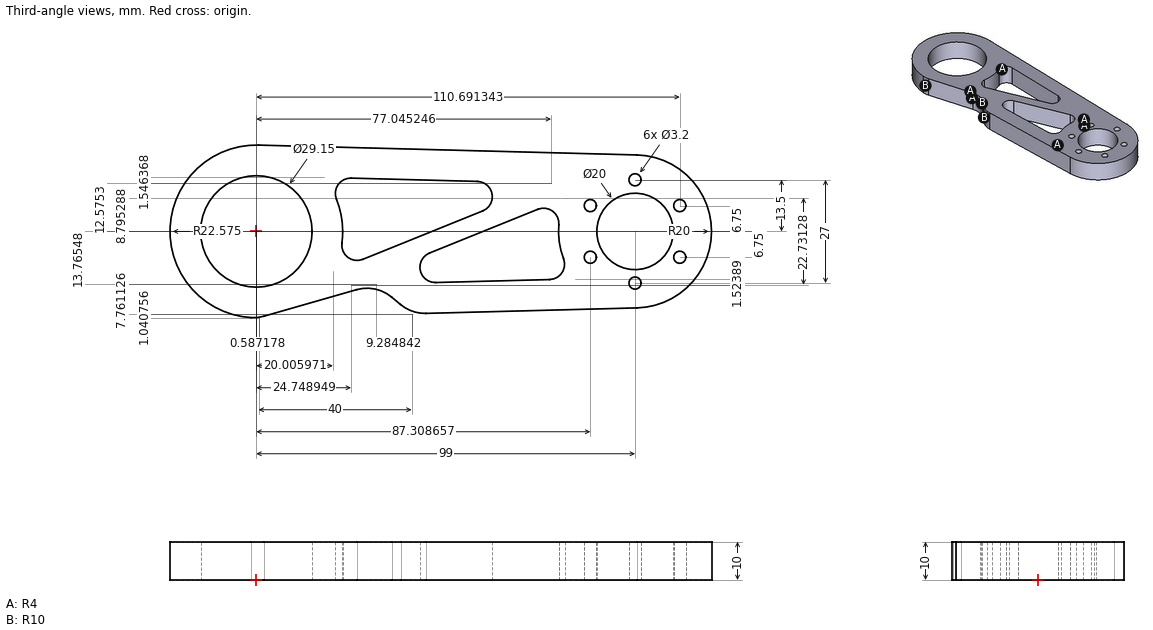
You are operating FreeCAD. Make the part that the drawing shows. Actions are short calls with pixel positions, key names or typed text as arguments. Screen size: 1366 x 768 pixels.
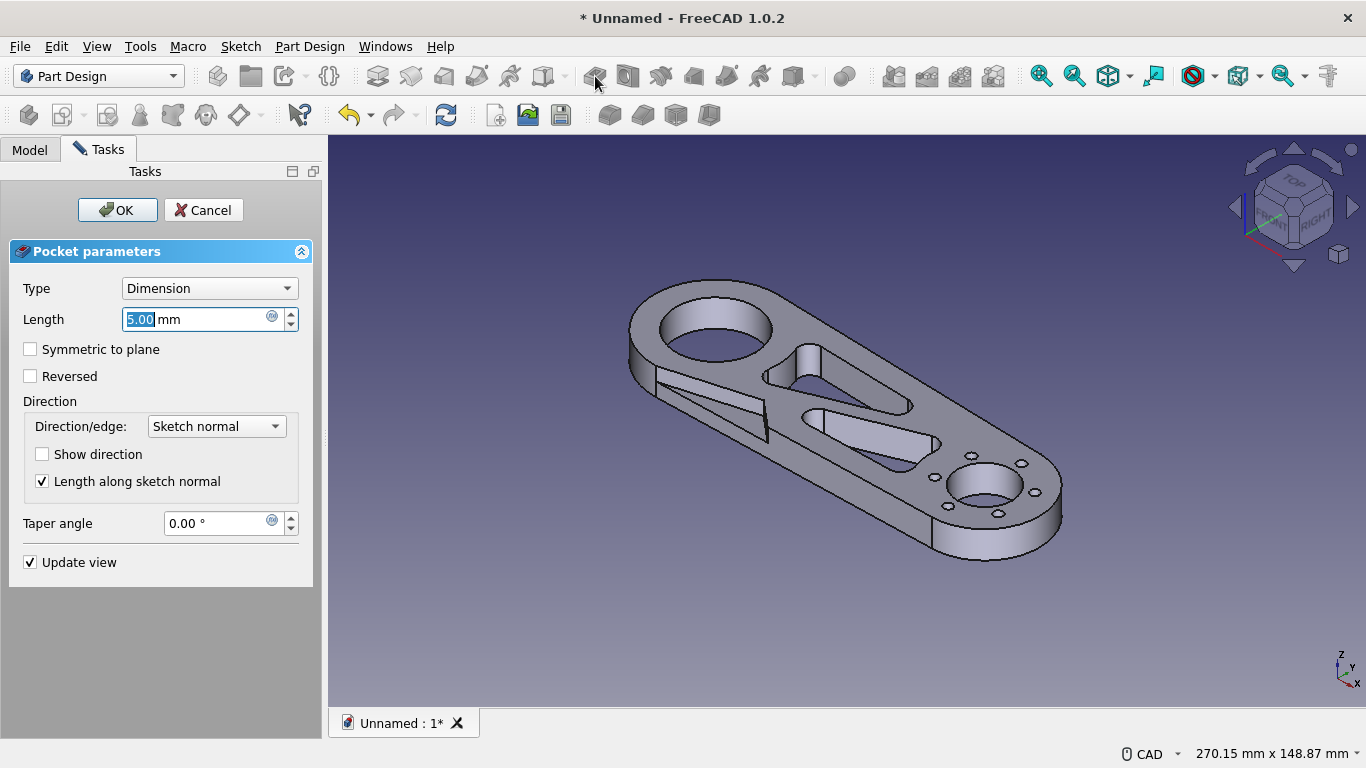
text(10)
key(Tab)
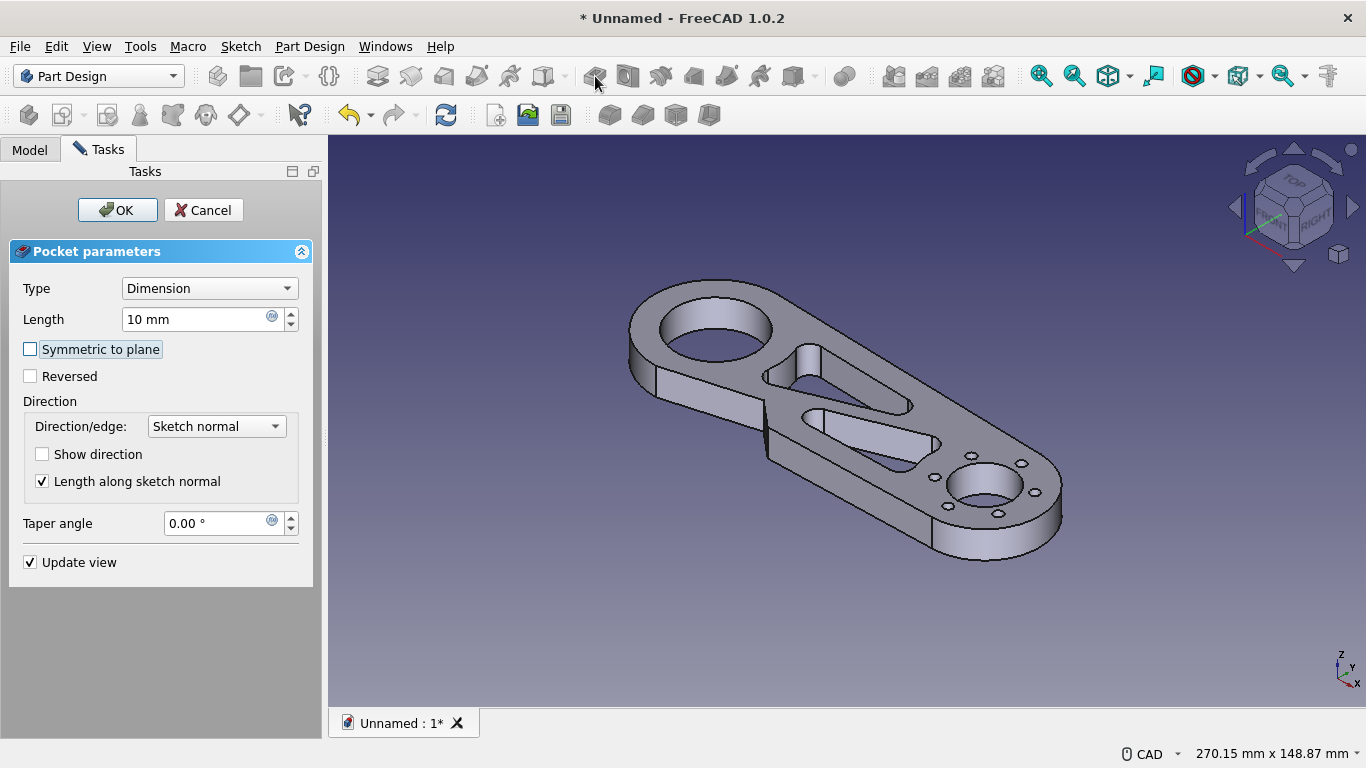
click(118, 210)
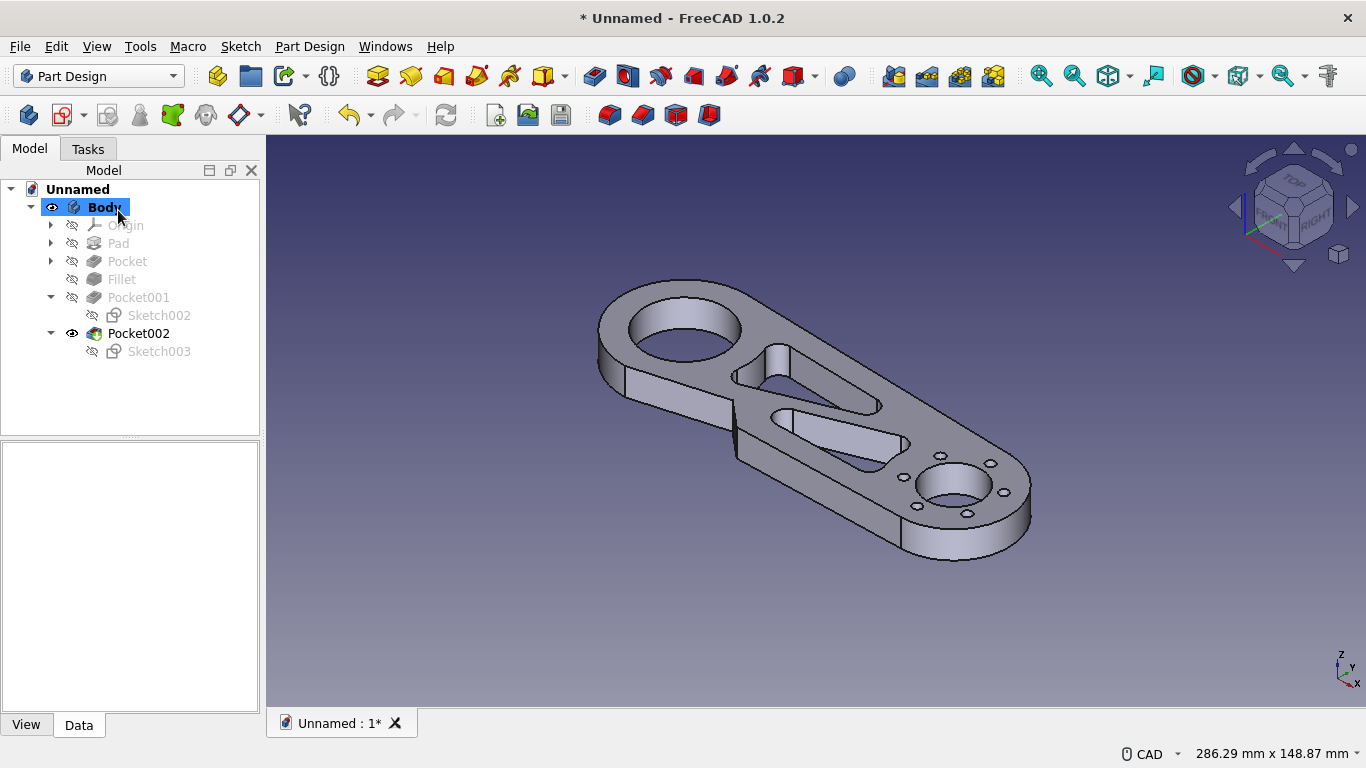
key(2)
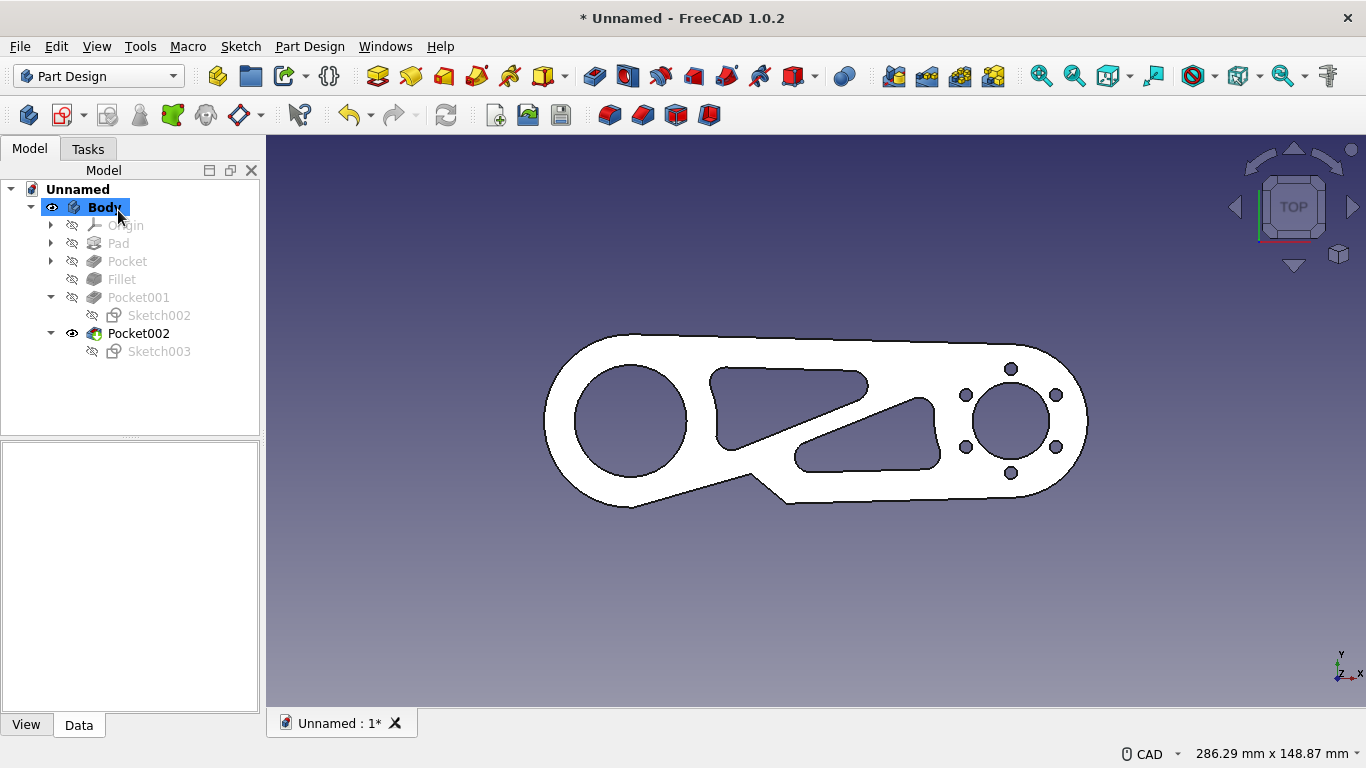
key(0)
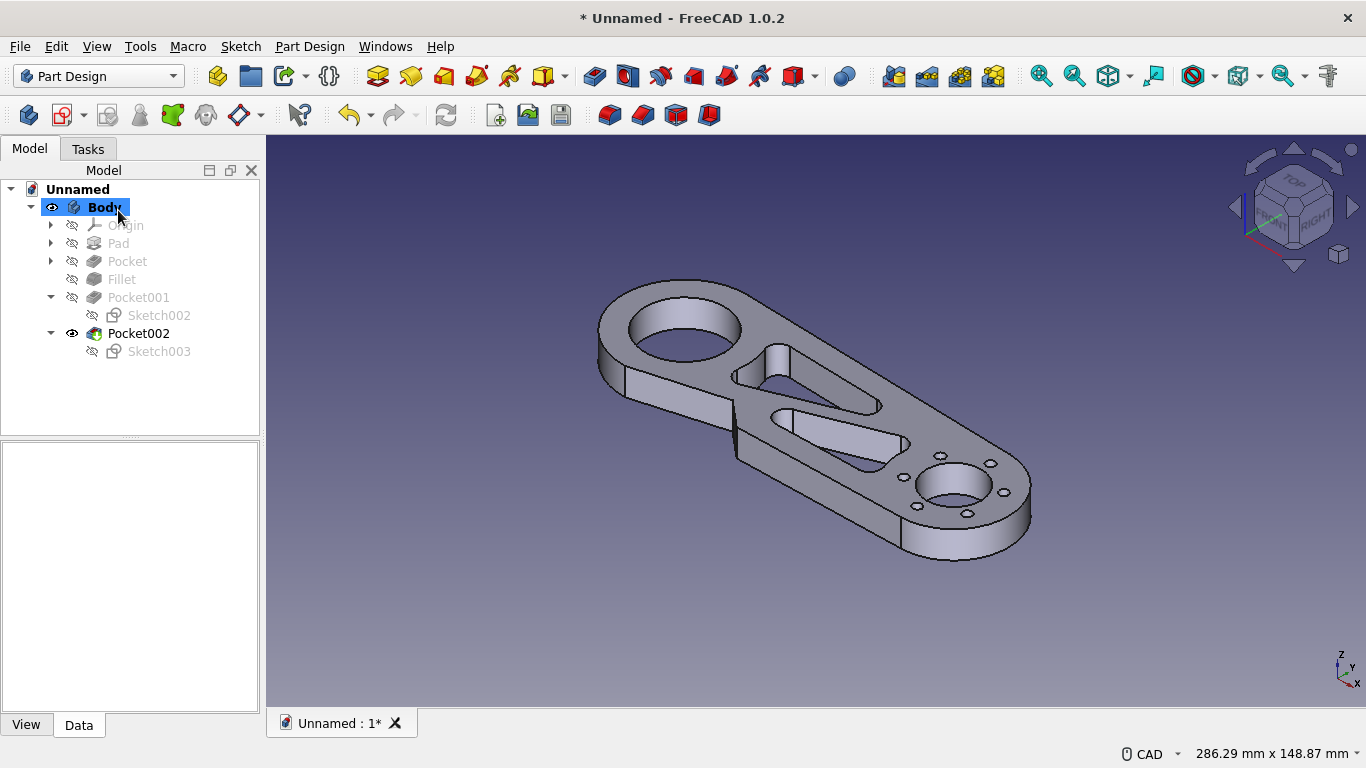
key(1)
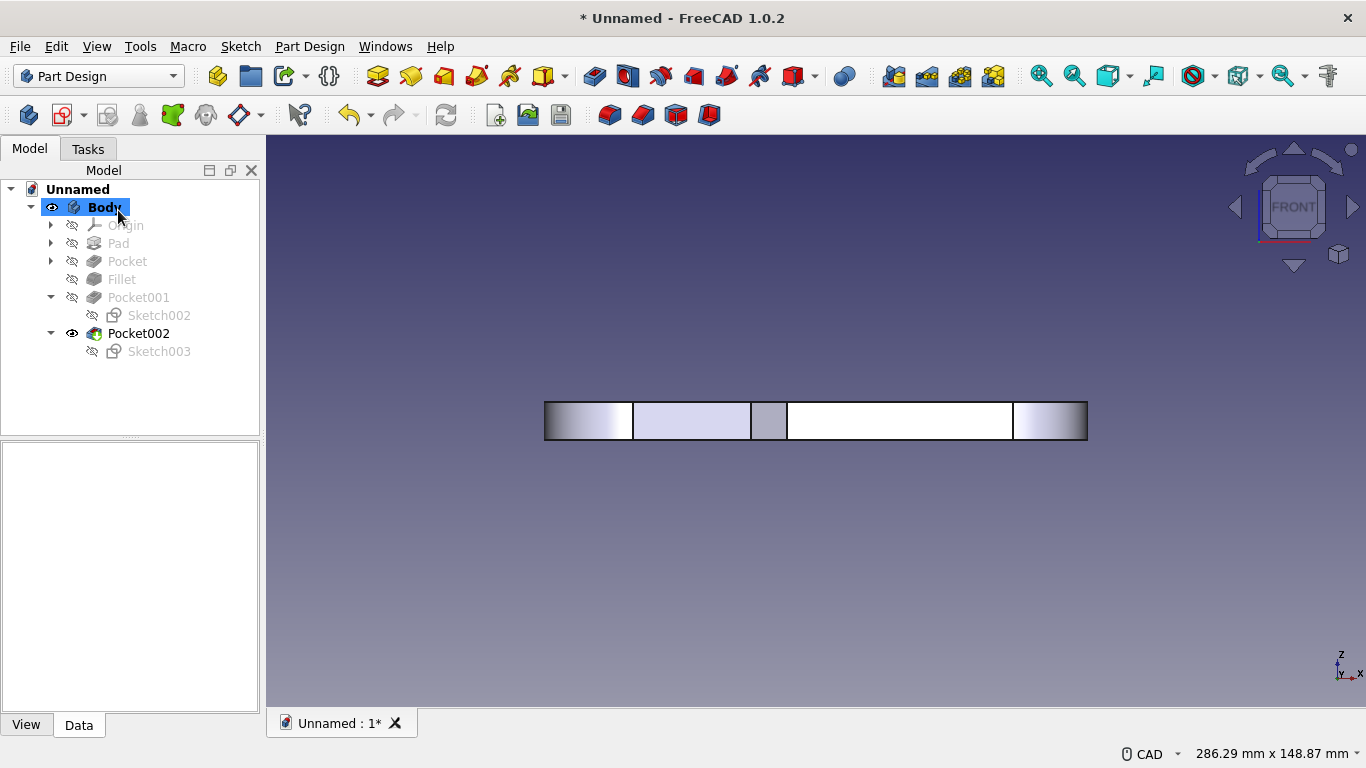
click(633, 420)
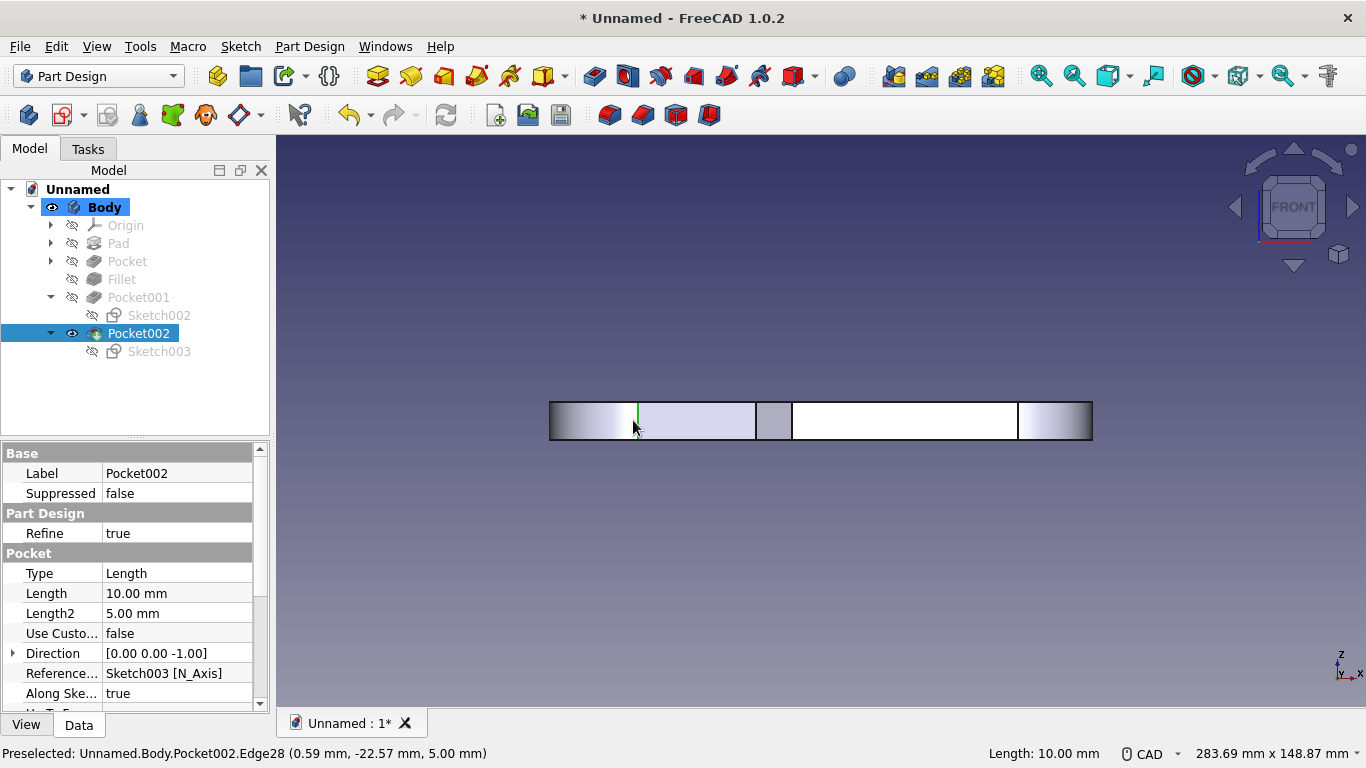
click(792, 420, ctrl)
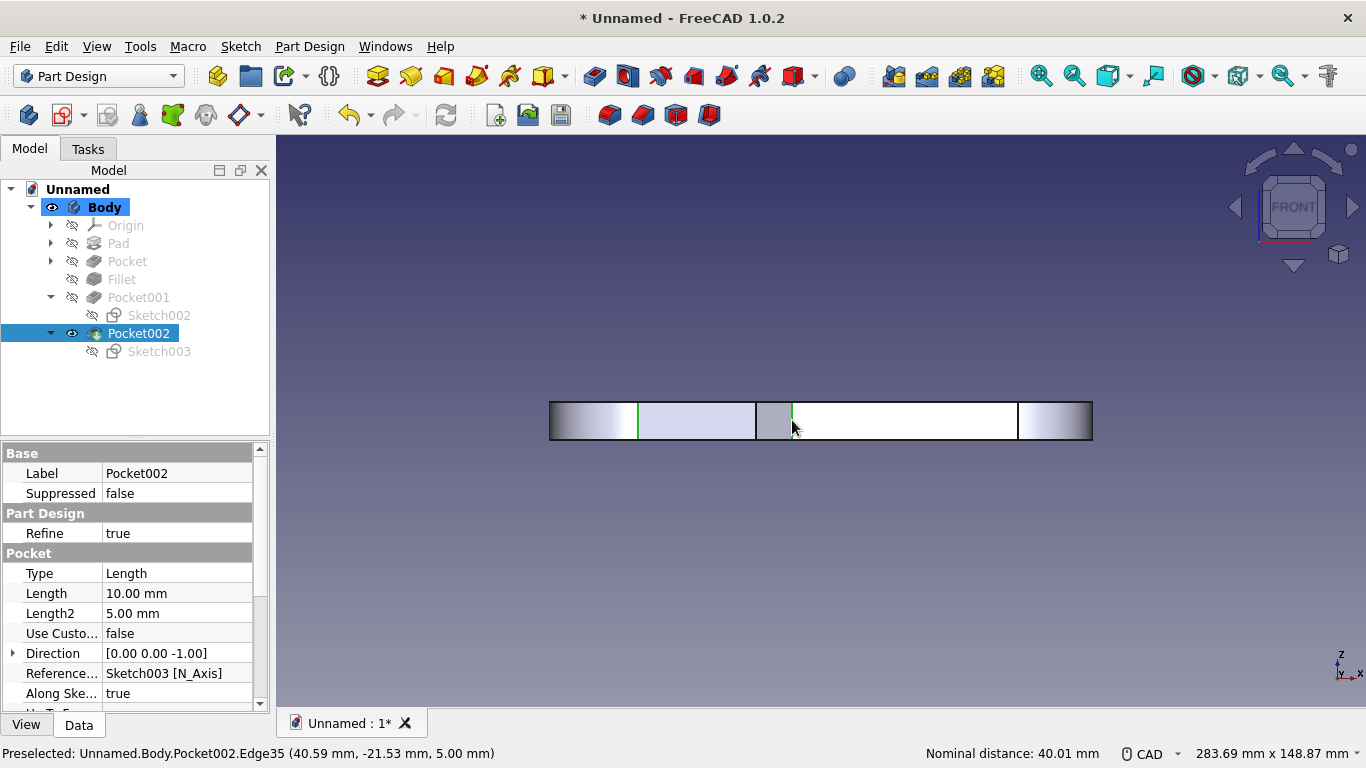
key(3)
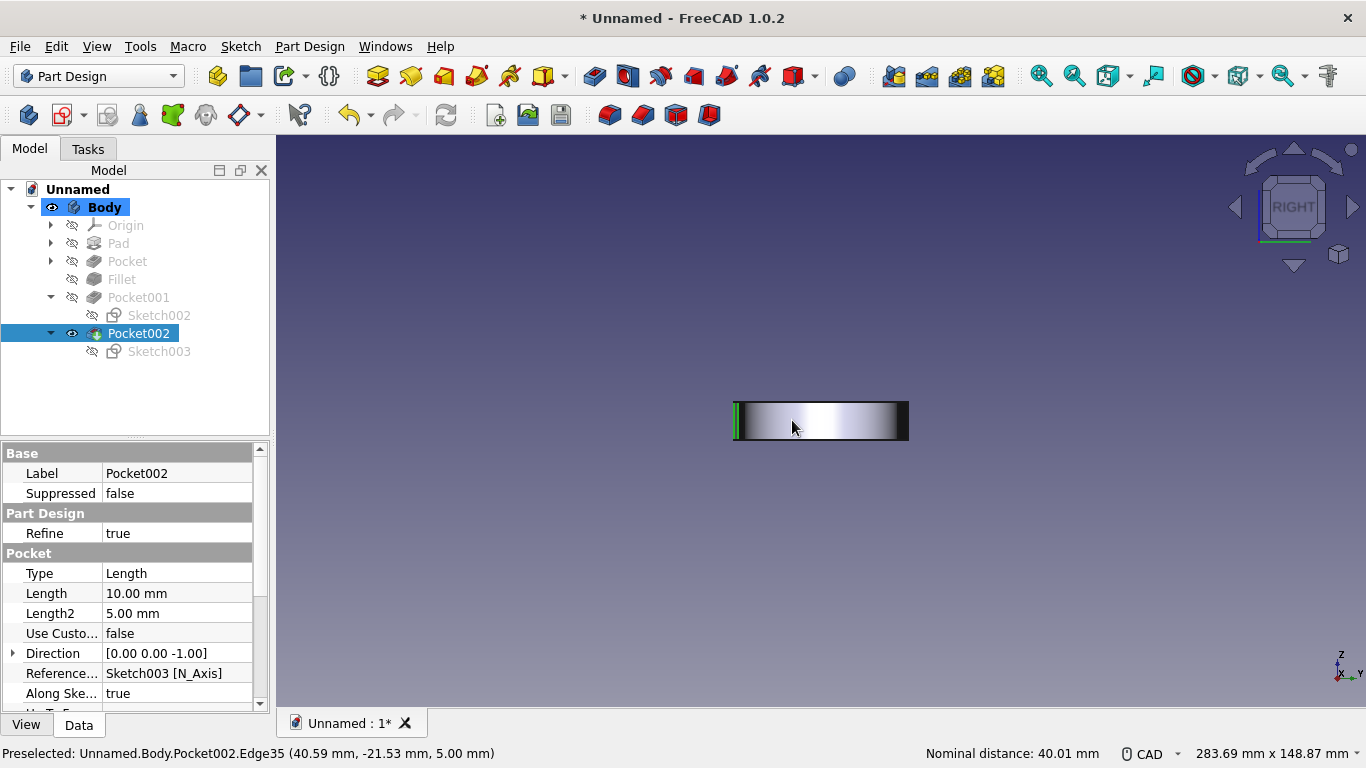
click(1042, 76)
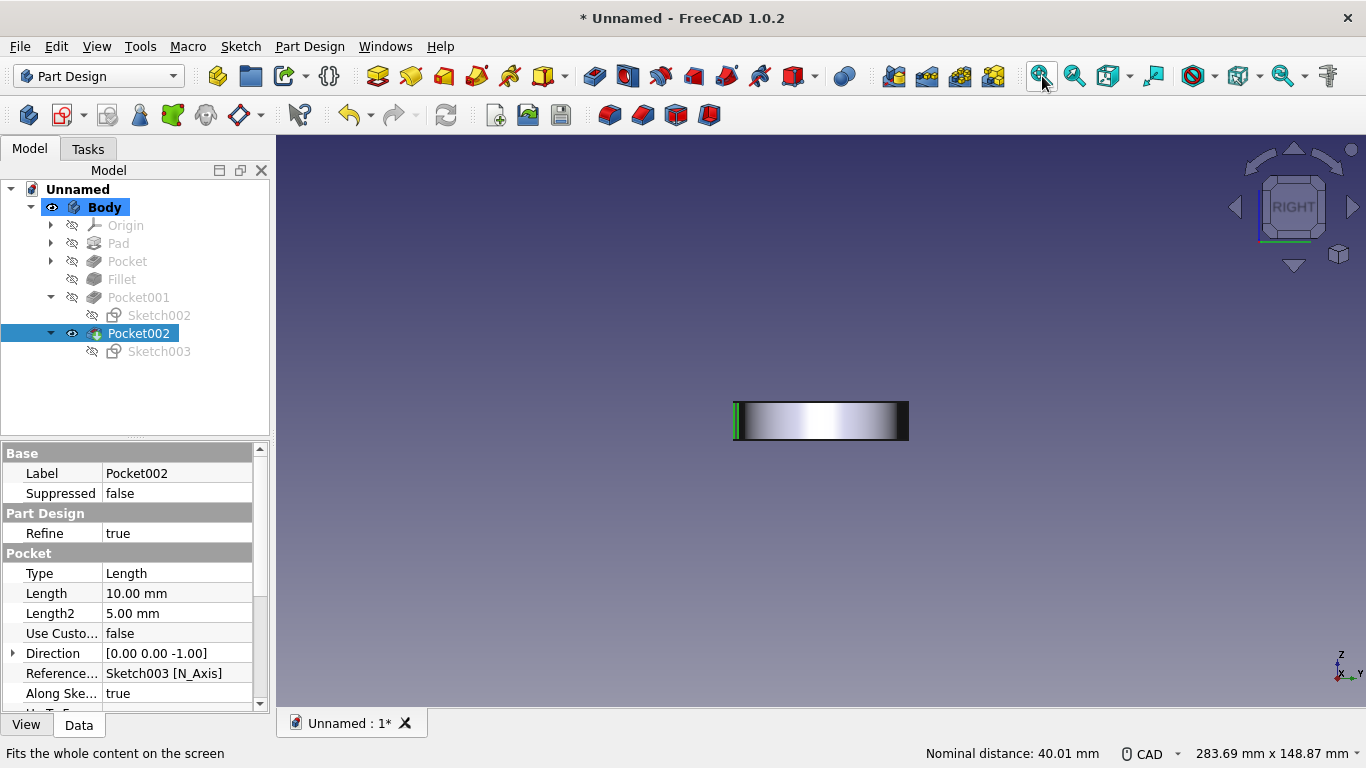
key(5)